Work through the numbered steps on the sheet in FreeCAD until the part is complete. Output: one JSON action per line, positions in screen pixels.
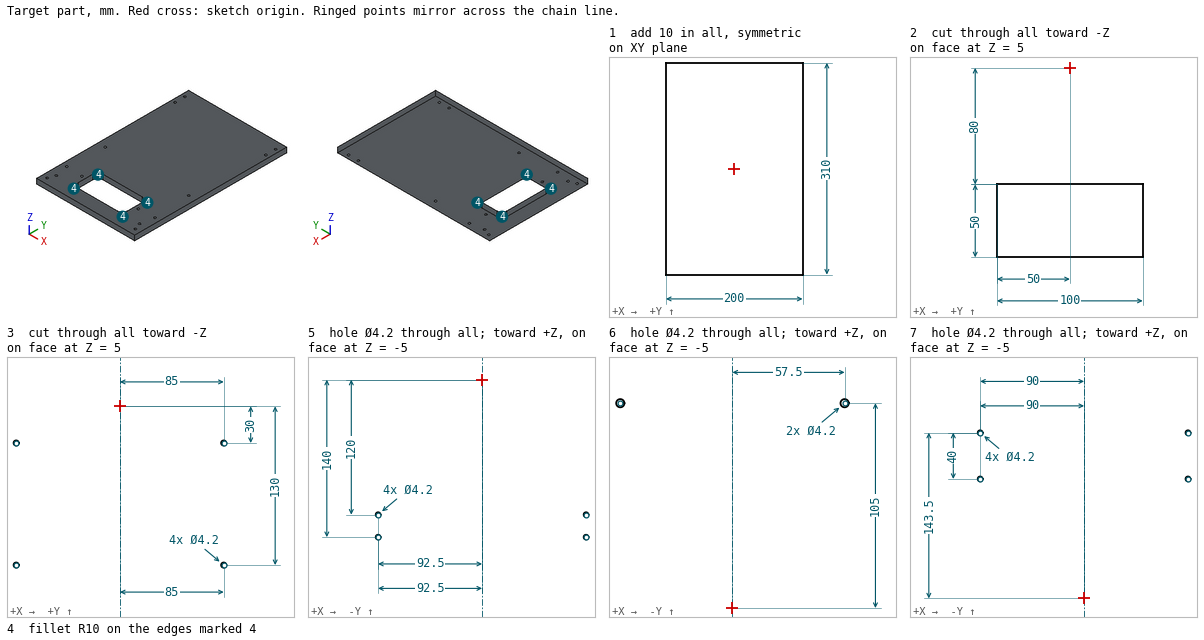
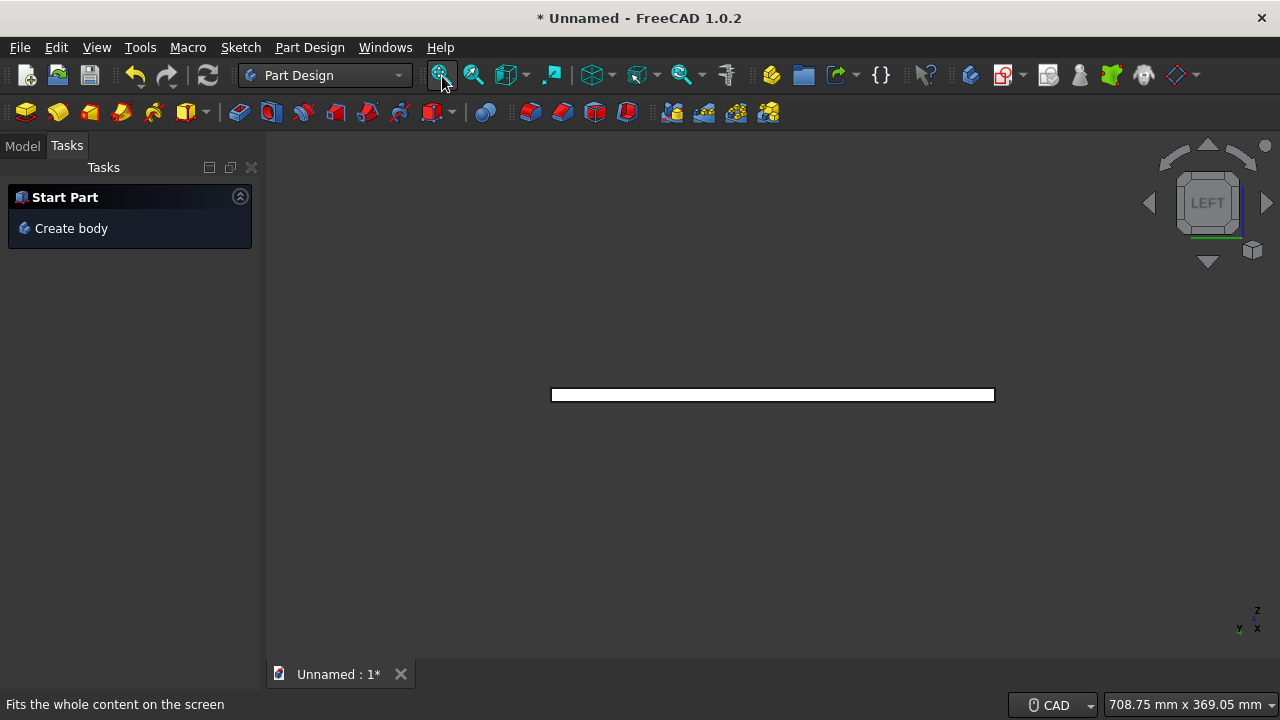
{"action": "key", "text": "0"}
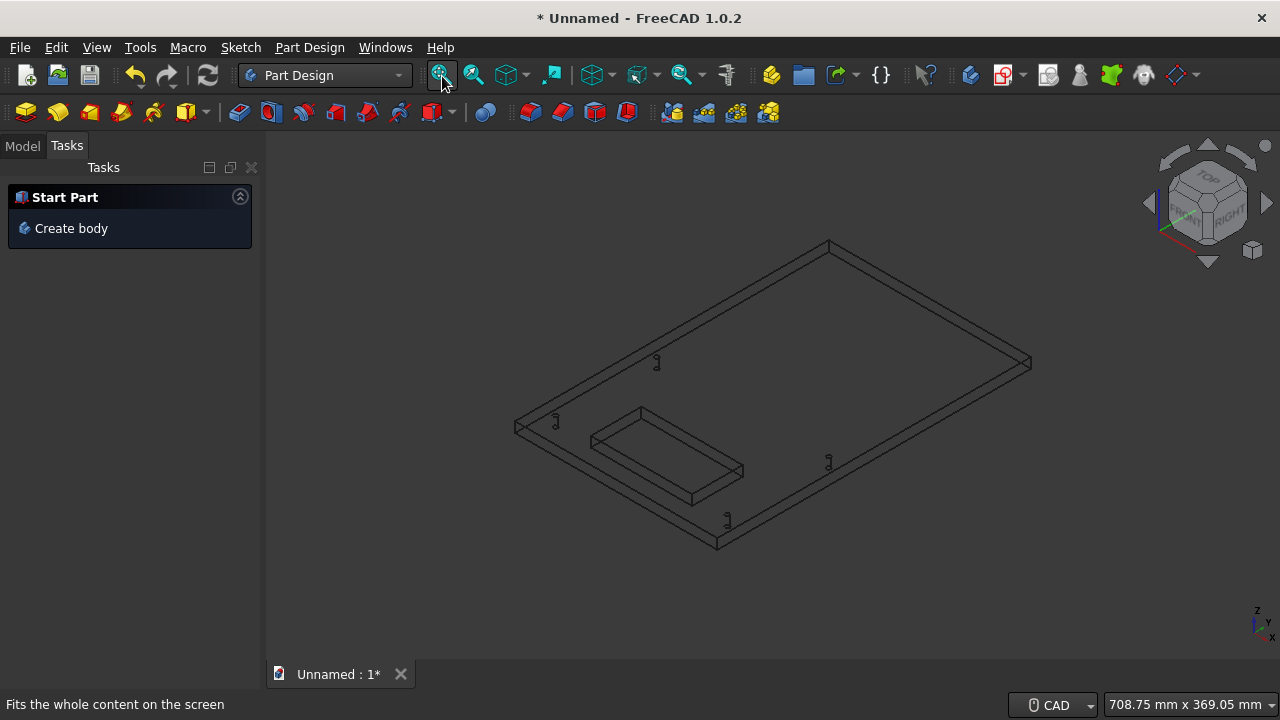
{"action": "left_click", "coordinate": [743, 472]}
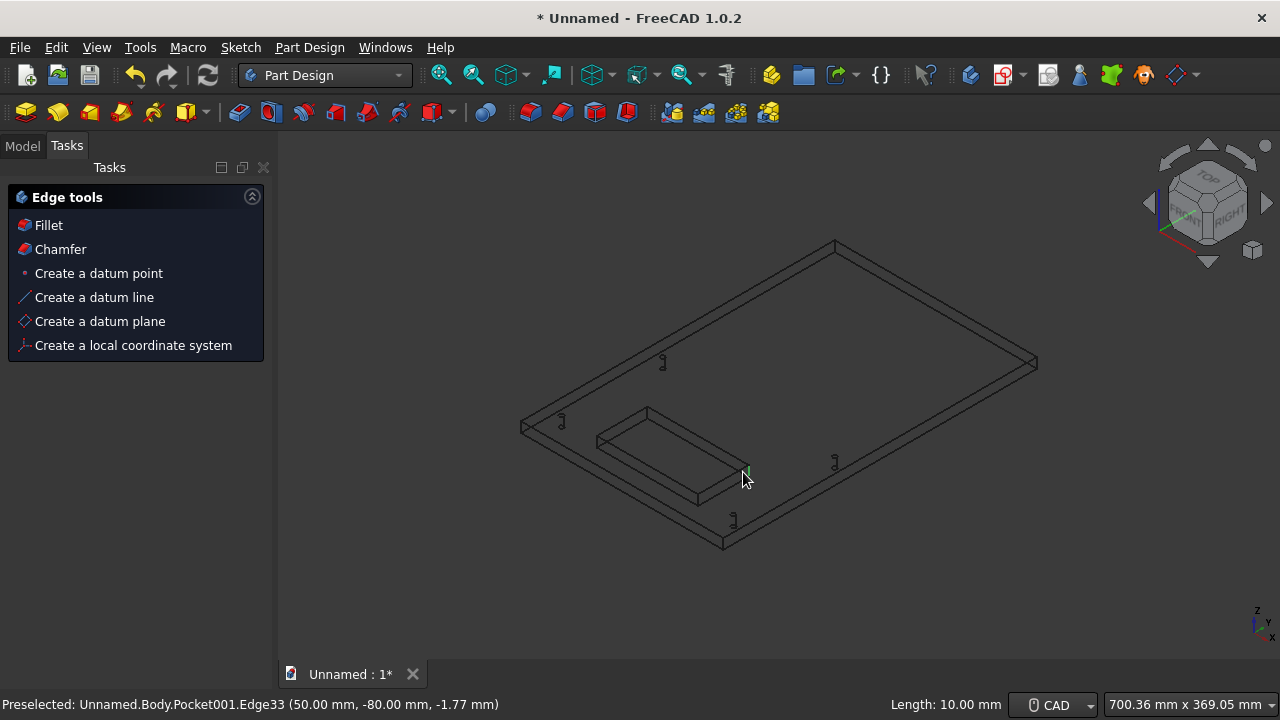
{"action": "left_click", "coordinate": [698, 500], "text": "ctrl"}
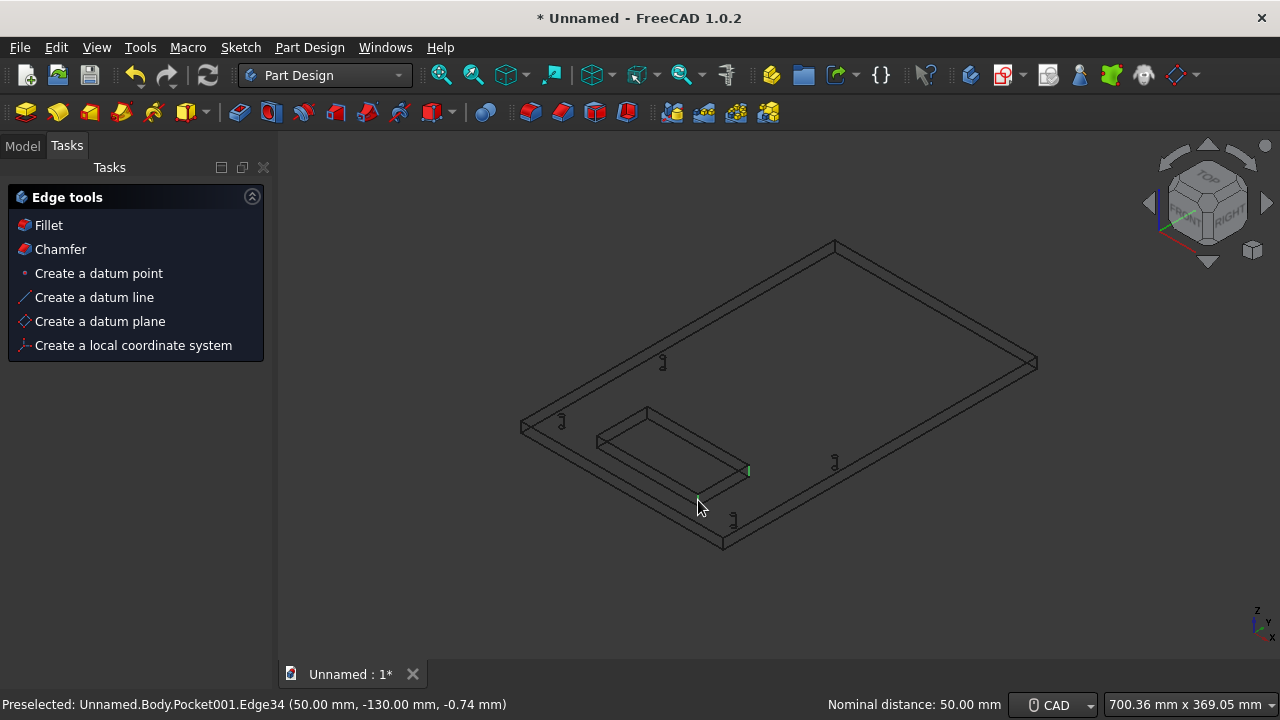
{"action": "left_click", "coordinate": [597, 443], "text": "ctrl"}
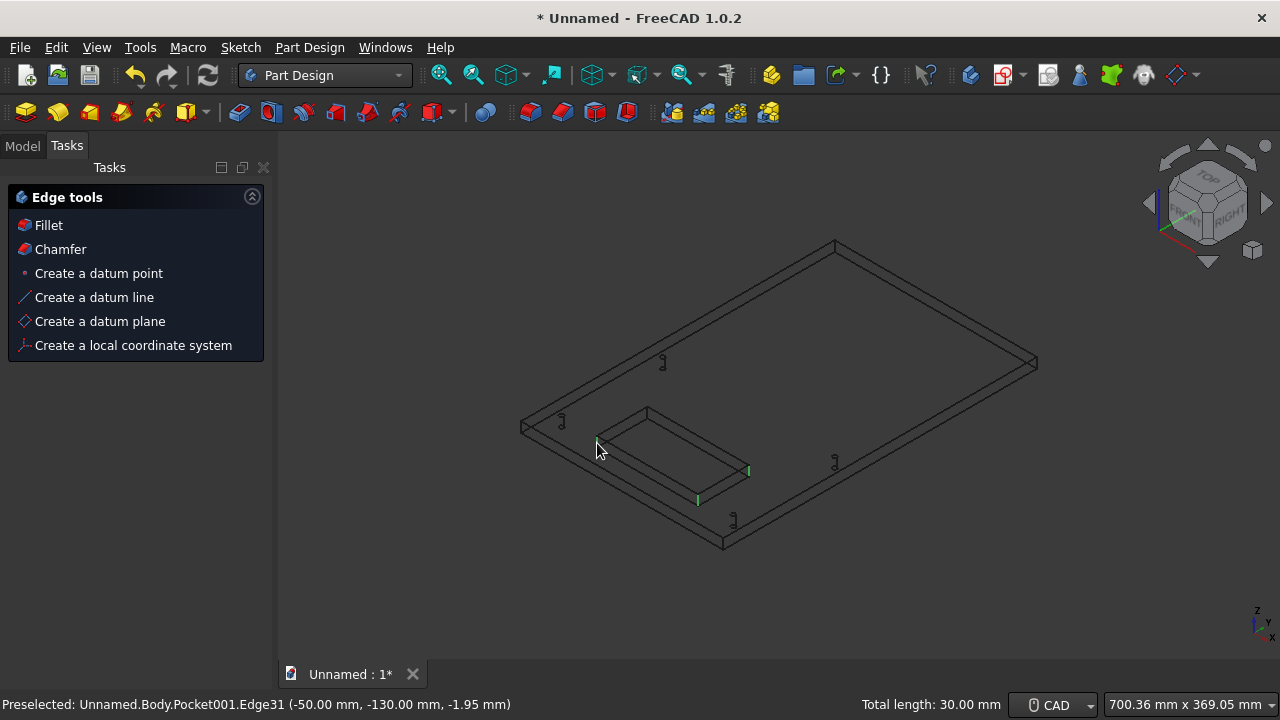
{"action": "left_click", "coordinate": [647, 414], "text": "ctrl"}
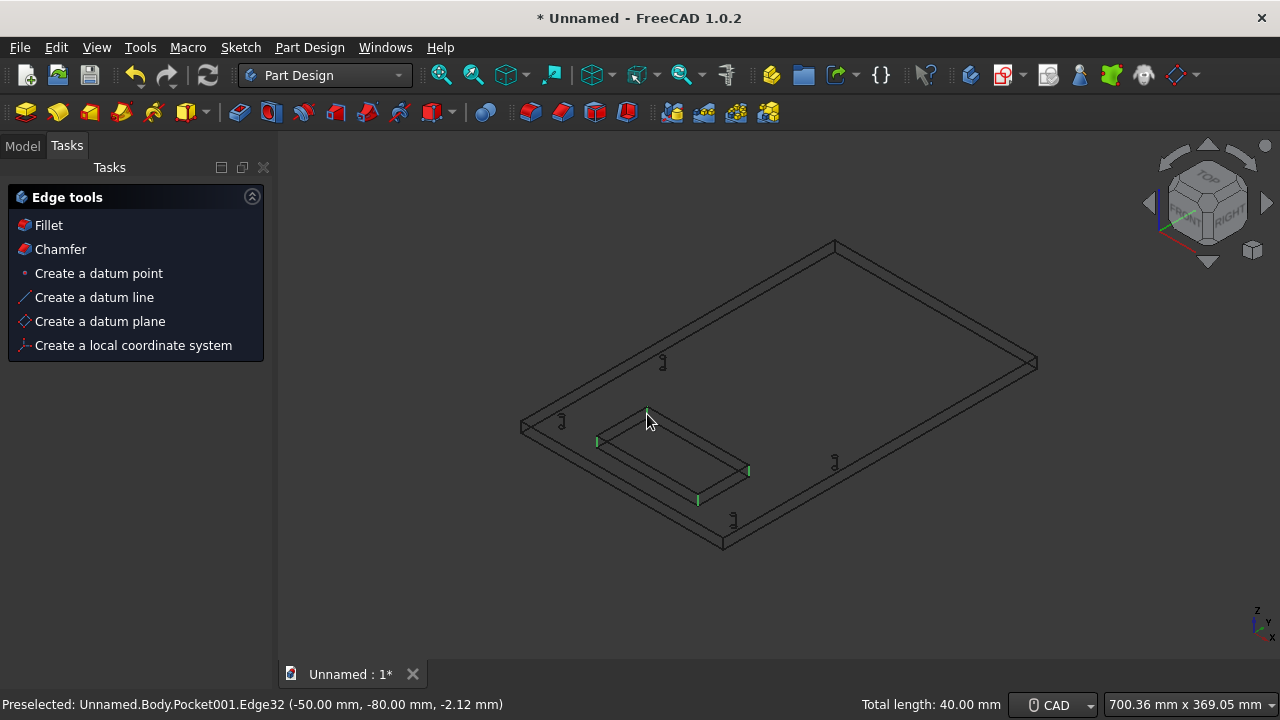
{"action": "key", "text": "v 1"}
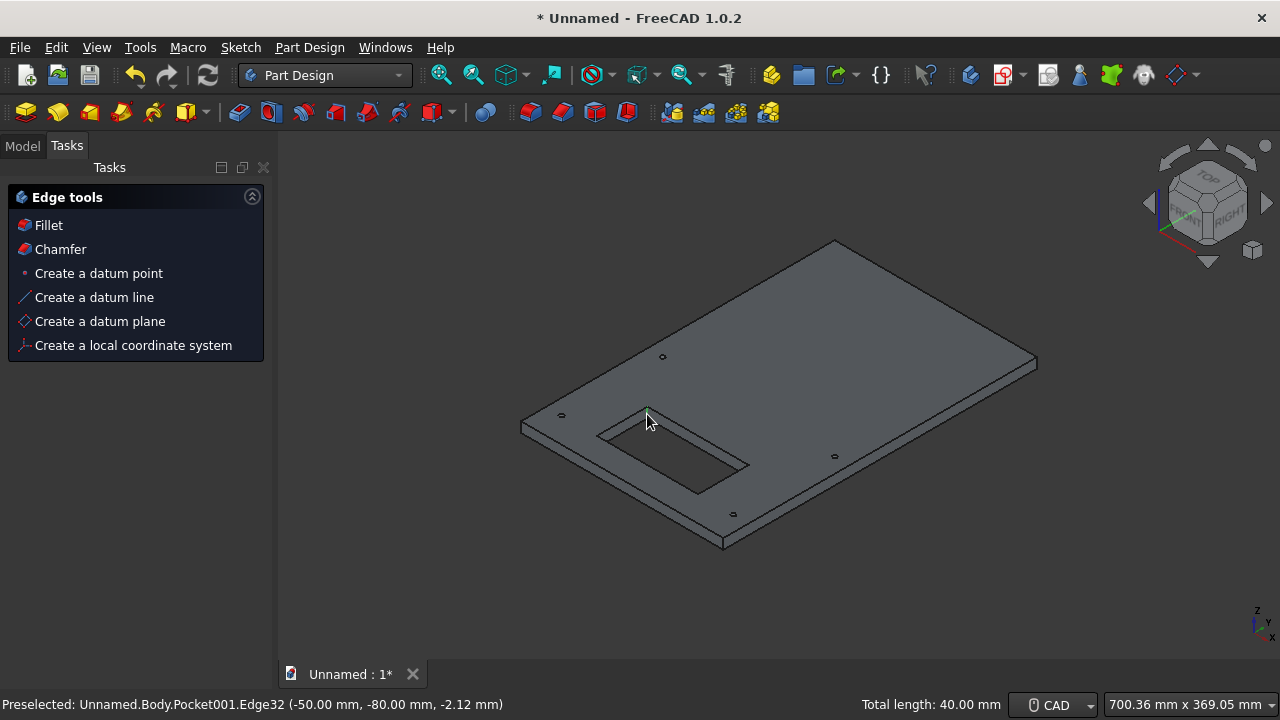
{"action": "left_click", "coordinate": [532, 112]}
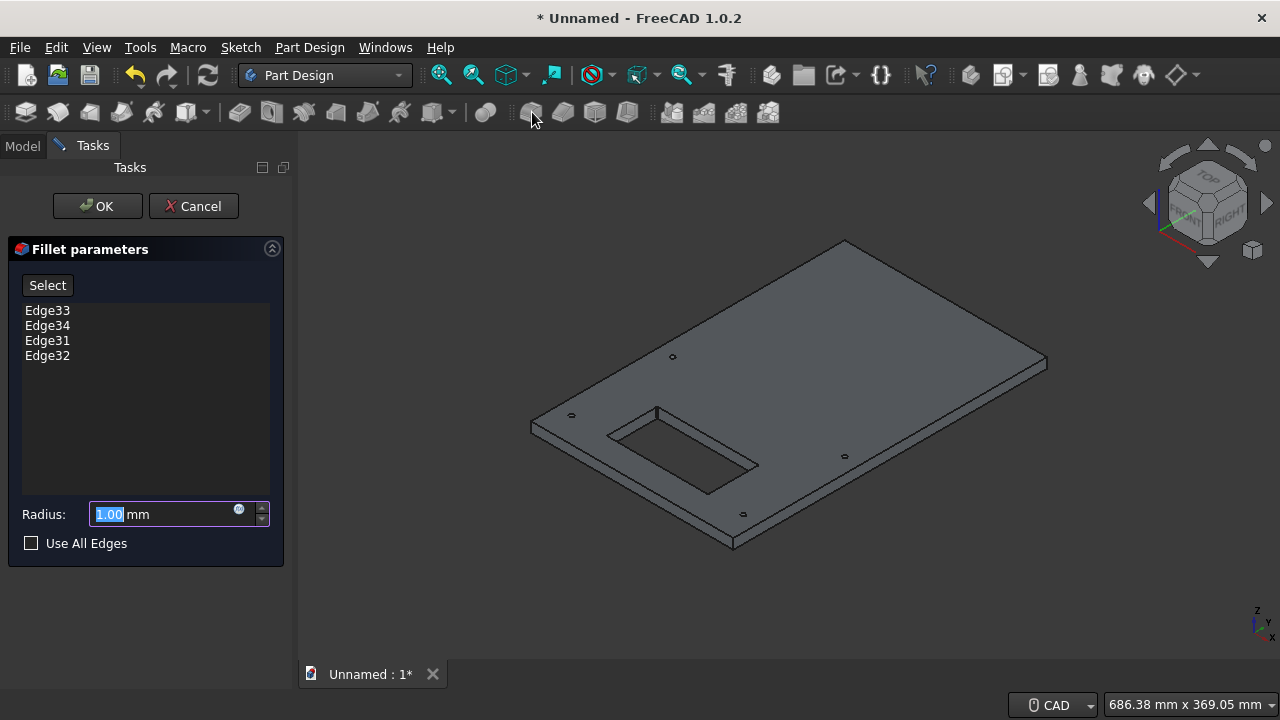
{"action": "type", "text": "10"}
{"action": "key", "text": "Tab"}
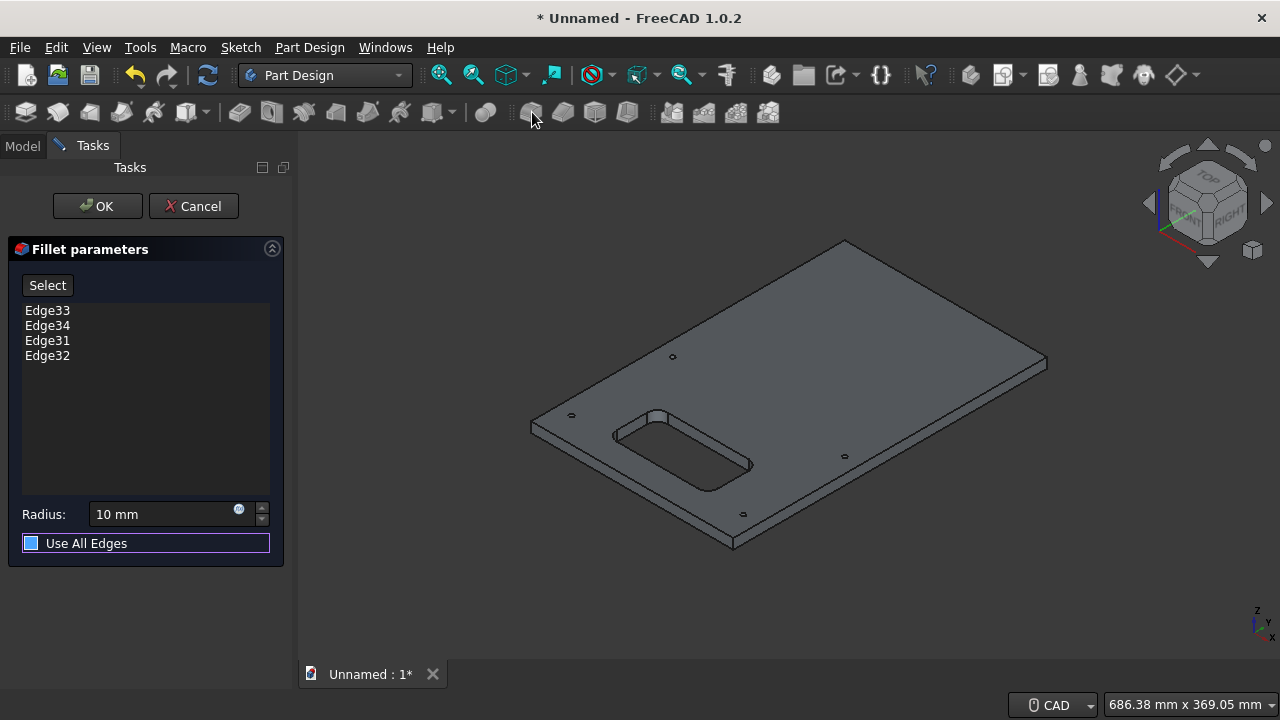
{"action": "left_click", "coordinate": [98, 206]}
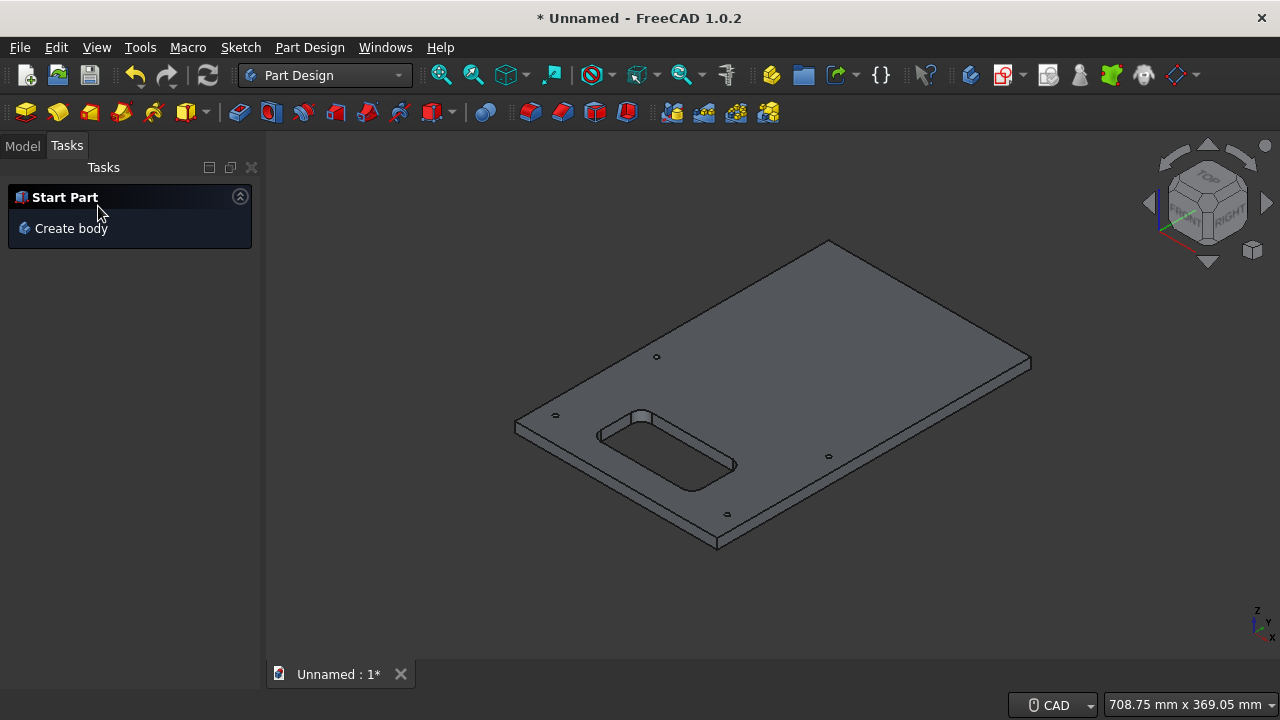
{"action": "key", "text": "5"}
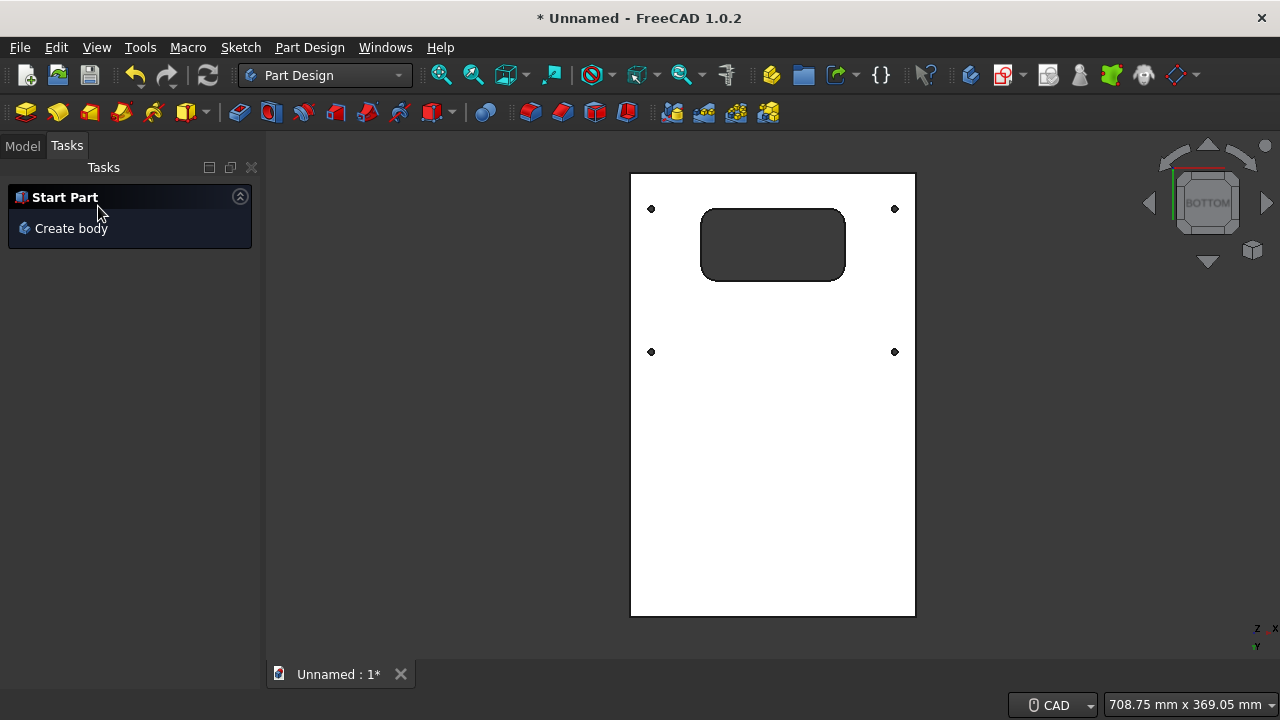
{"action": "left_click", "coordinate": [773, 457]}